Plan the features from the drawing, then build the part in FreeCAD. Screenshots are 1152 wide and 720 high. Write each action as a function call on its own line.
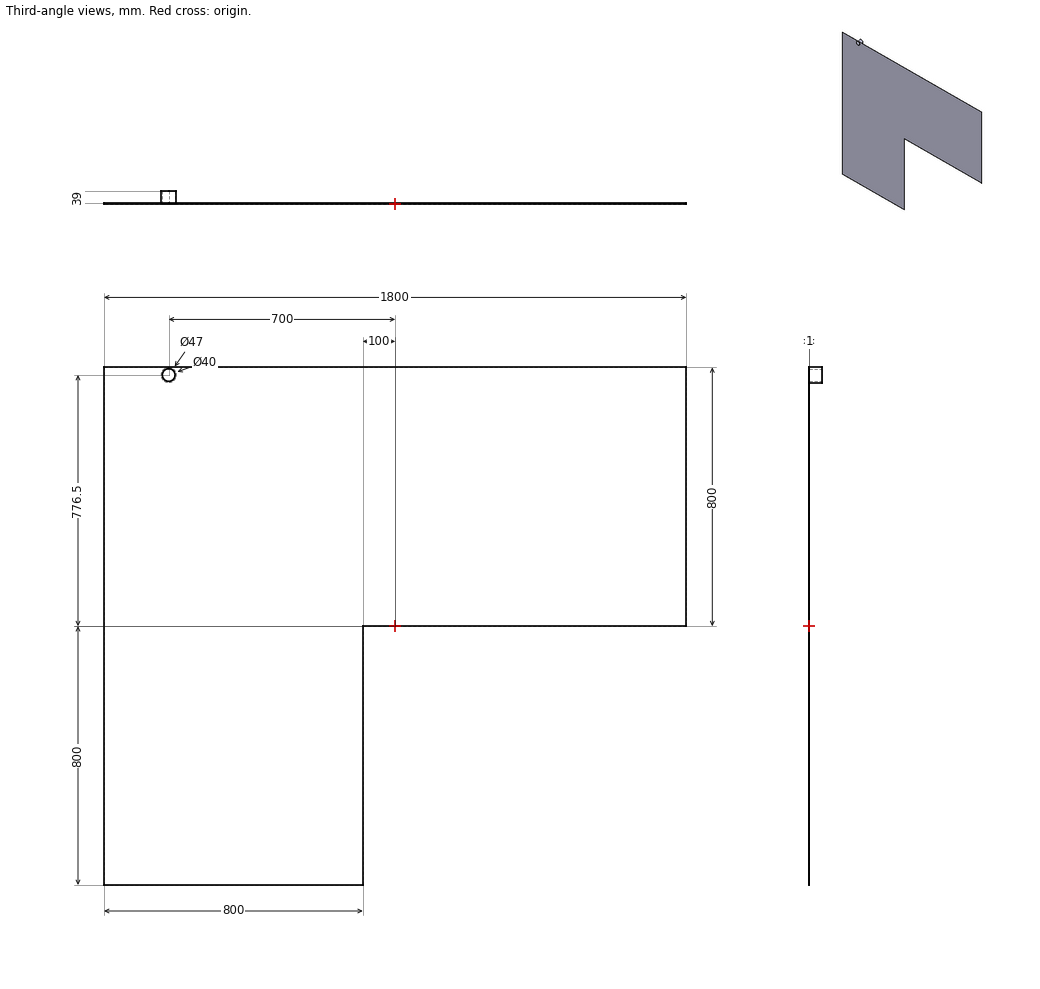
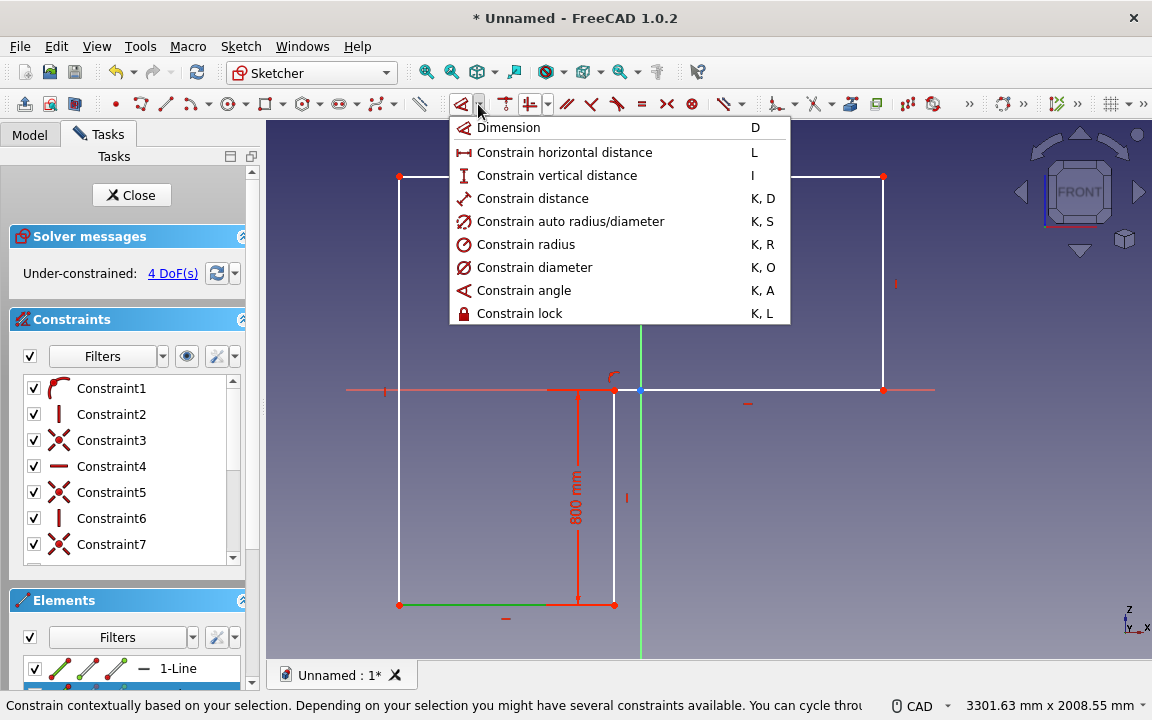
click(620, 152)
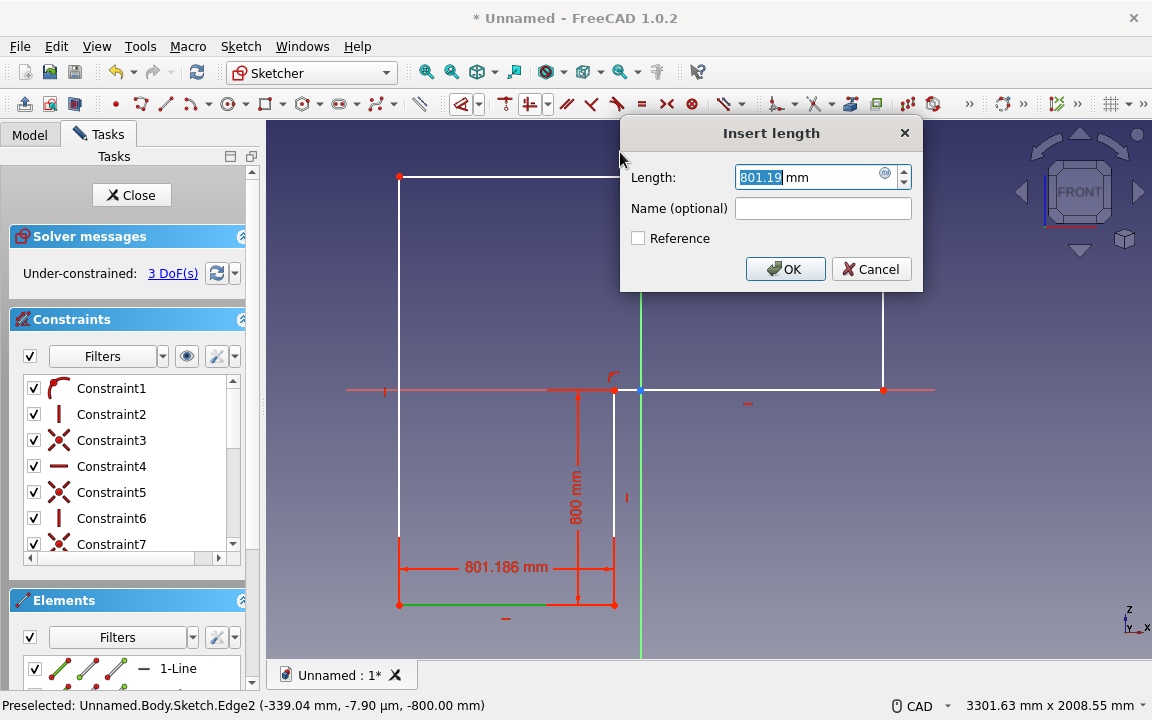
text(800)
key(Return)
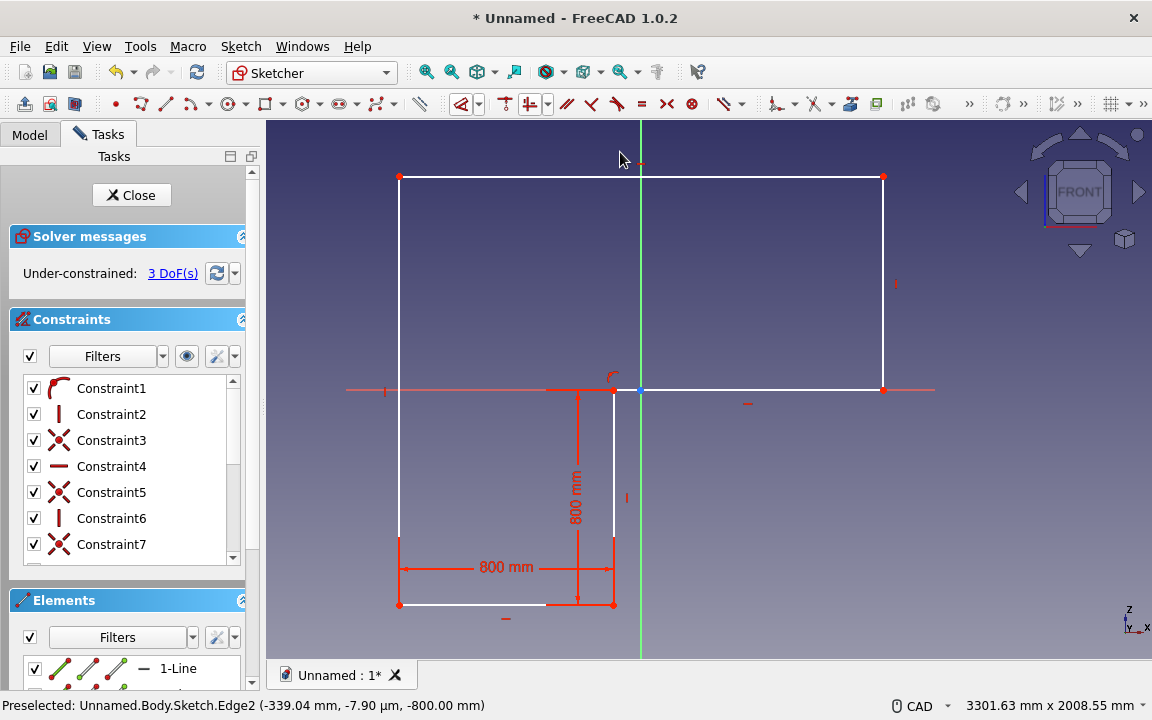
click(883, 241)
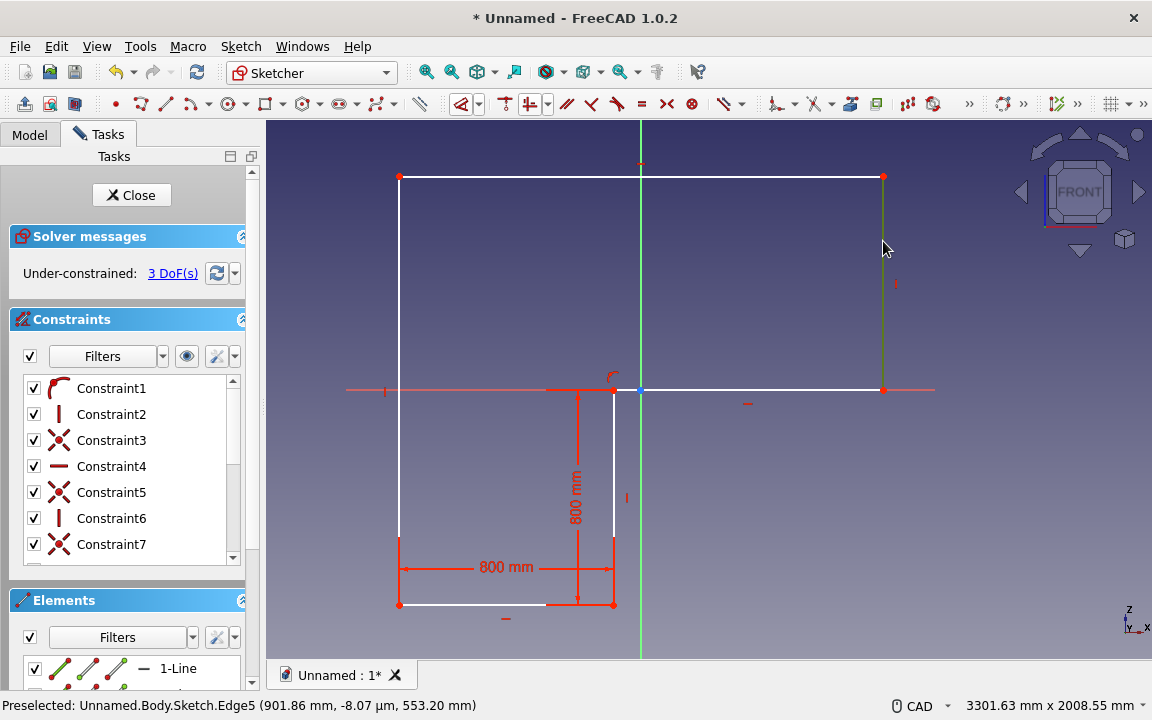
key(i)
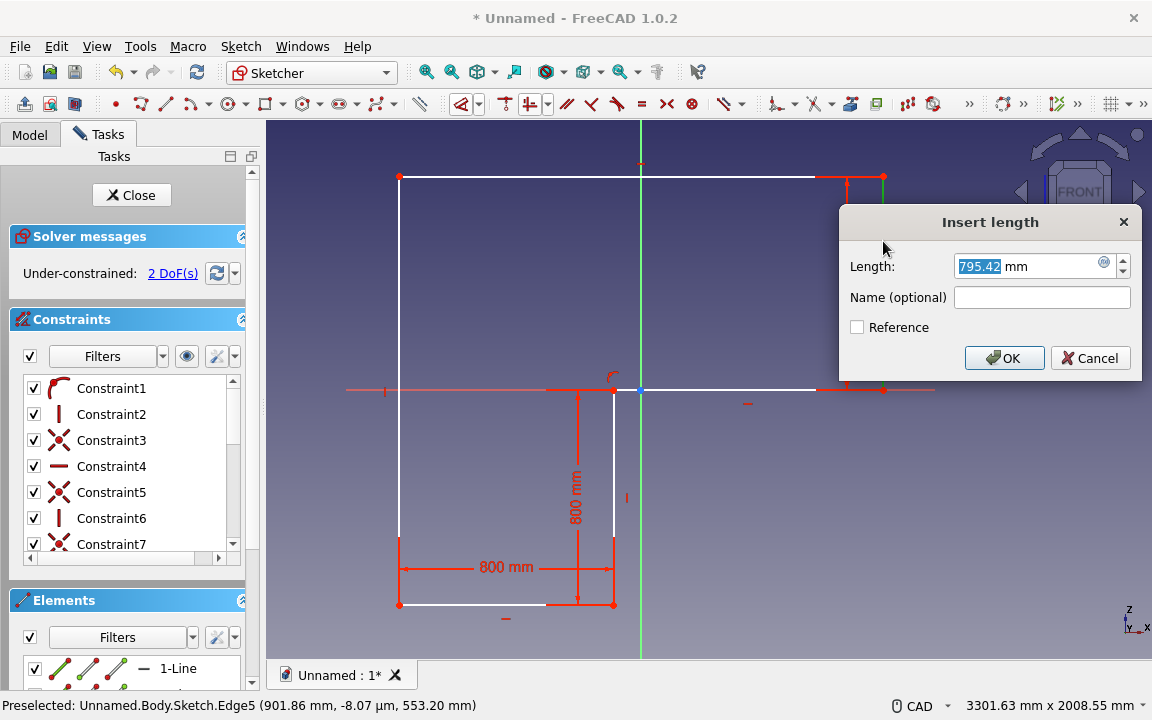
text(800)
key(Return)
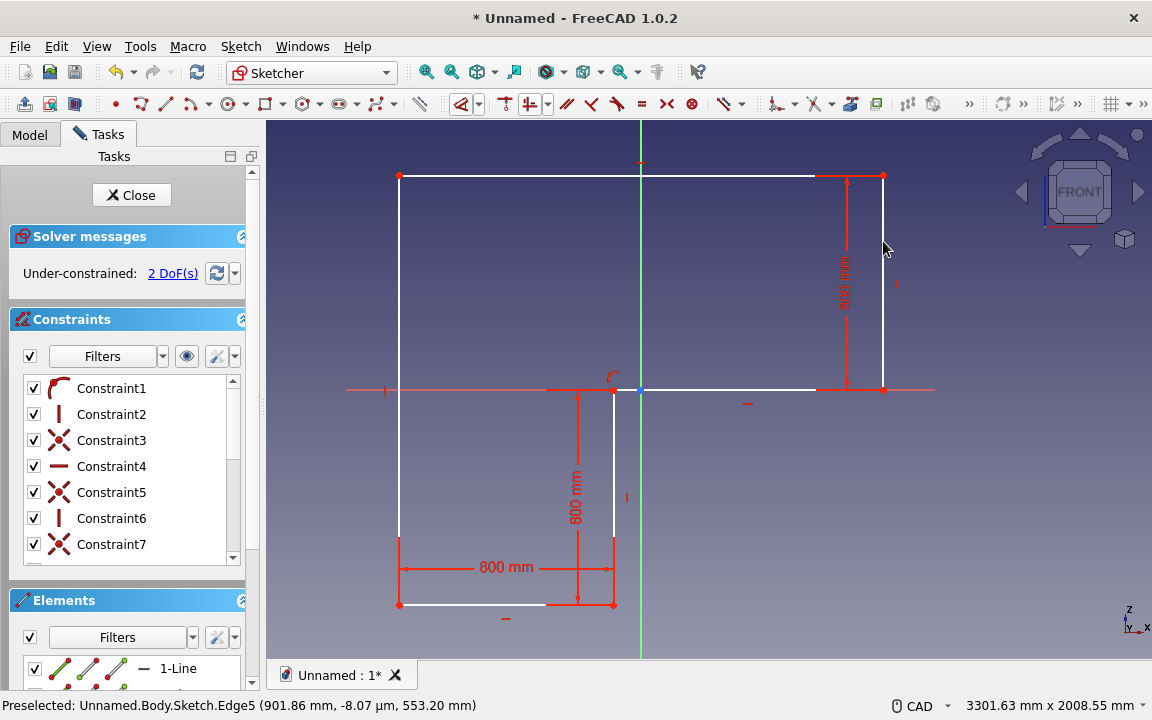
click(544, 176)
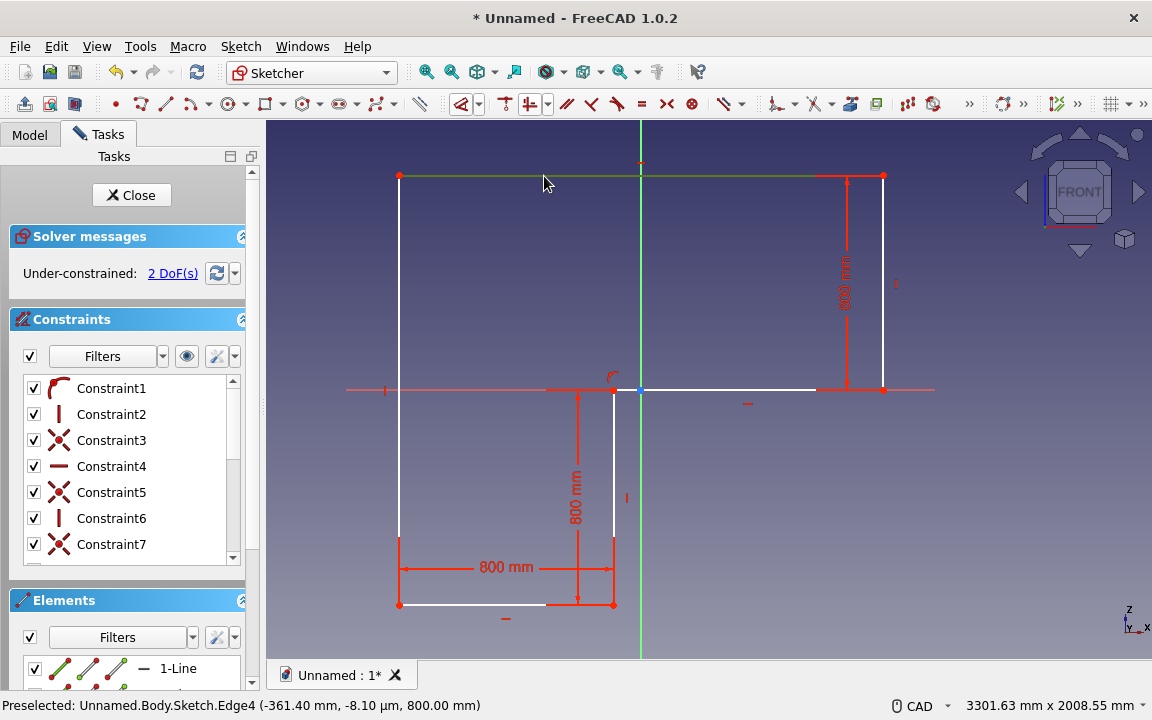
key(l)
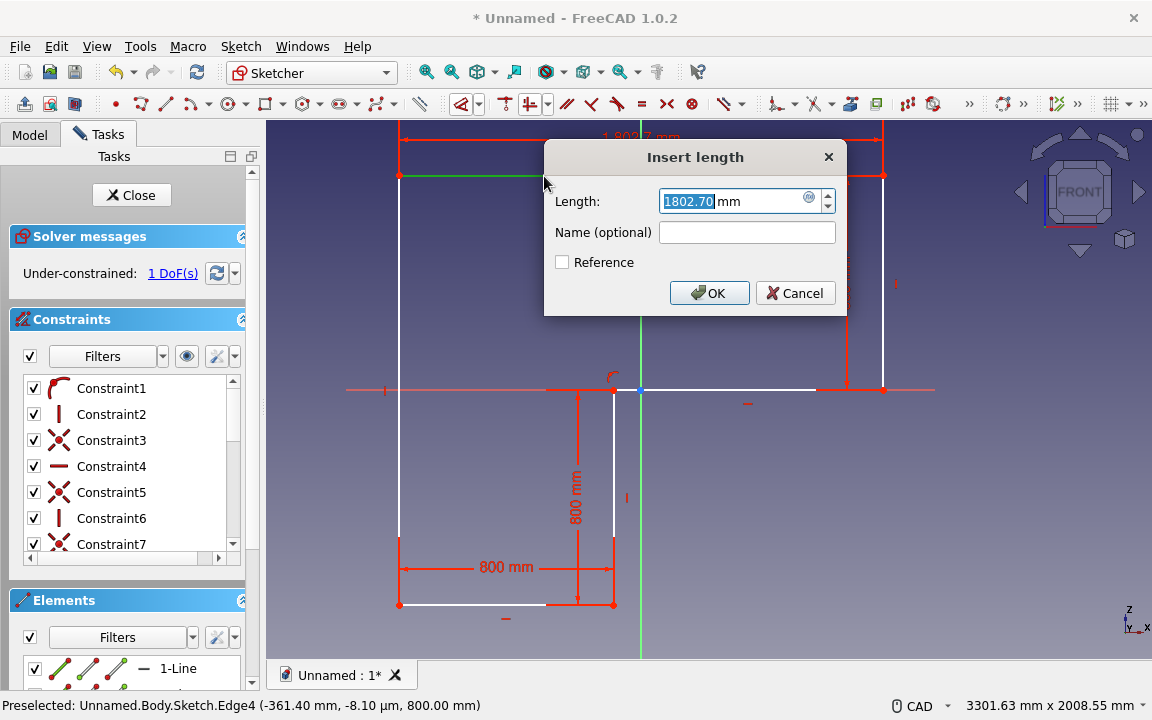
text(1800)
key(Return)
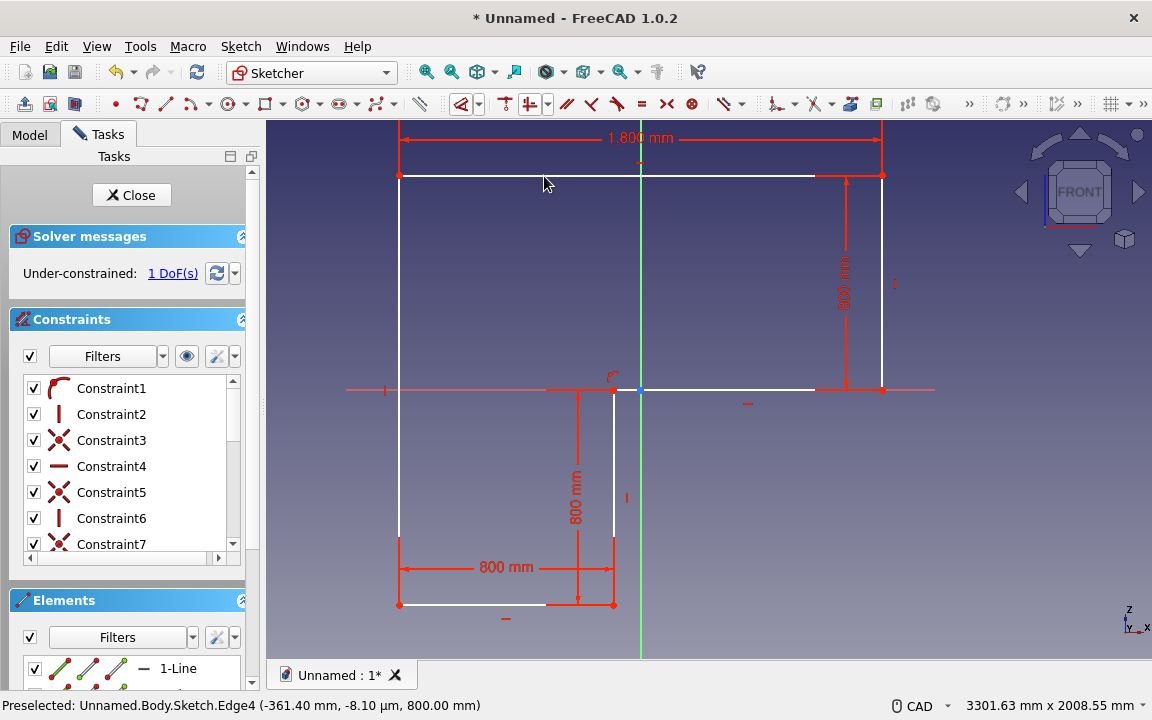
scroll(614, 390, up, 2)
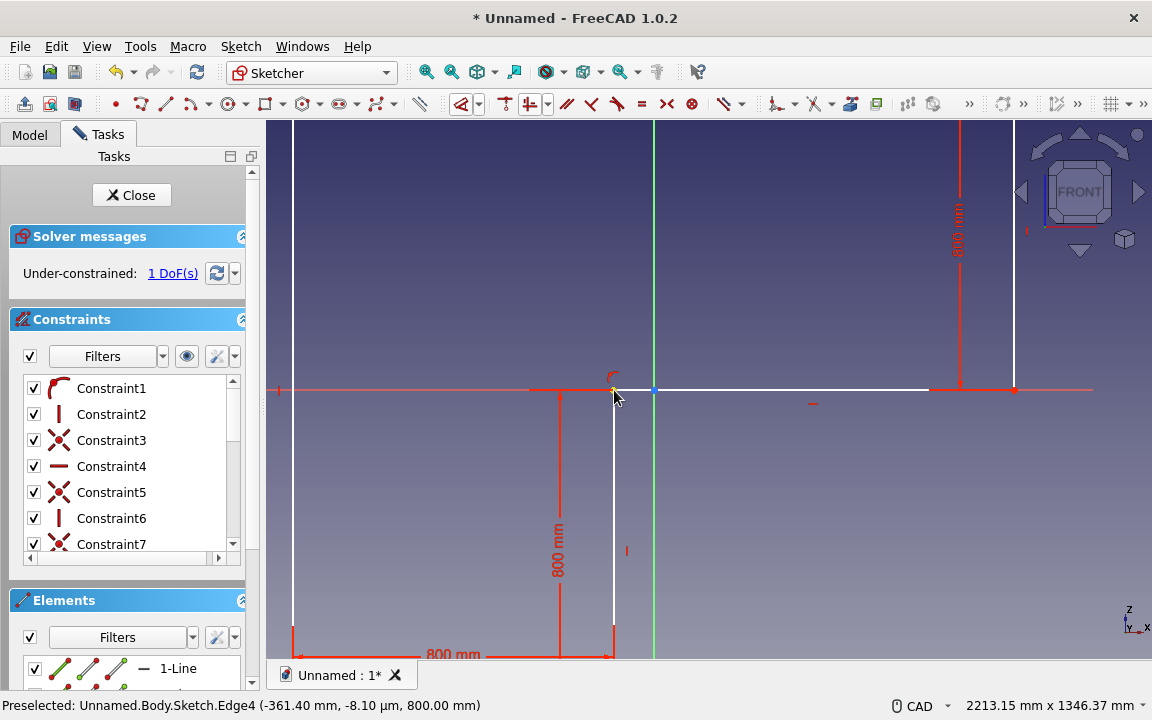
click(614, 390)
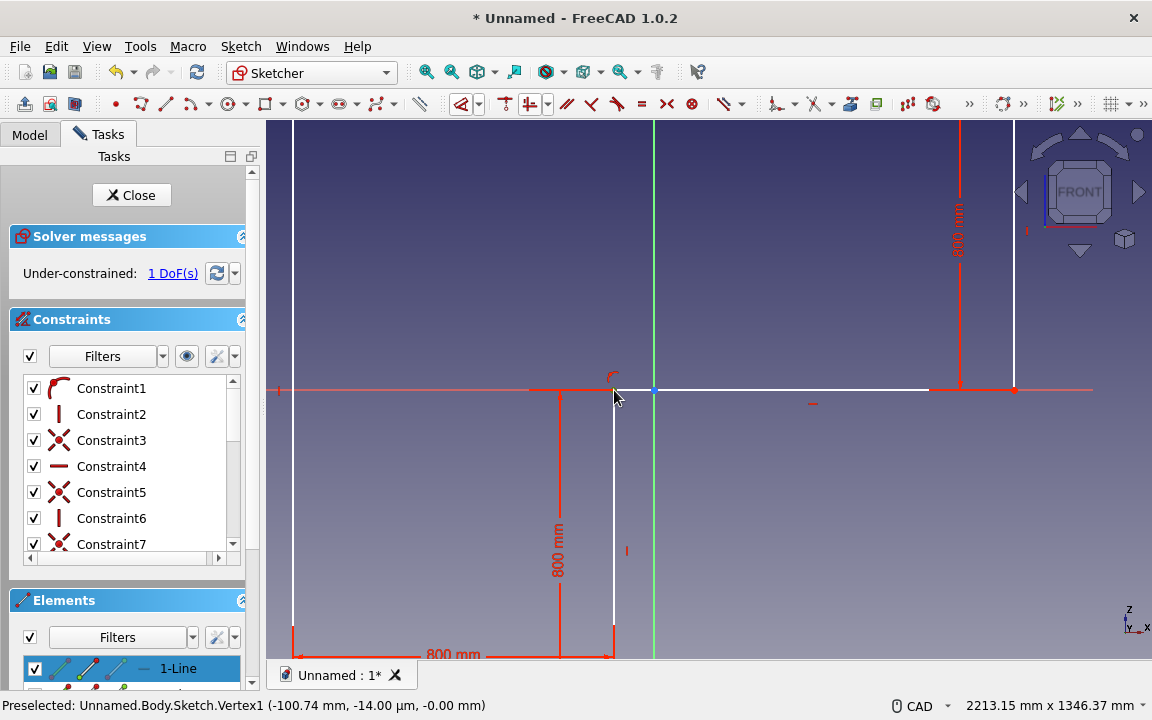
click(478, 104)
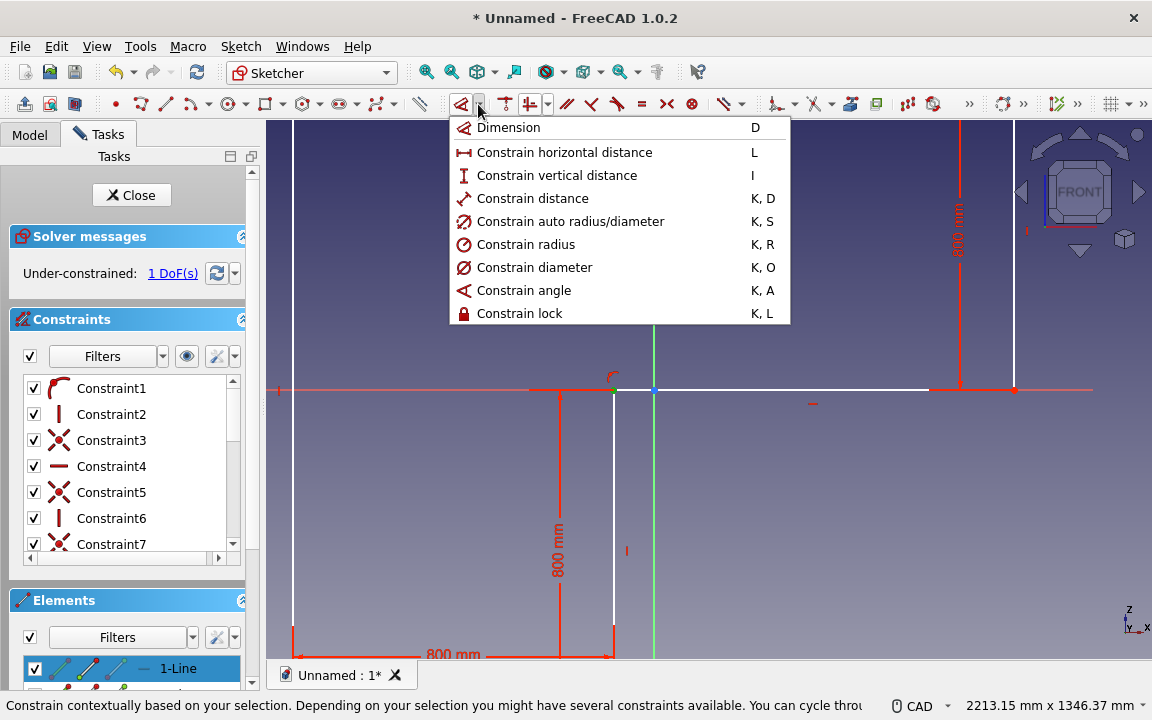
click(620, 152)